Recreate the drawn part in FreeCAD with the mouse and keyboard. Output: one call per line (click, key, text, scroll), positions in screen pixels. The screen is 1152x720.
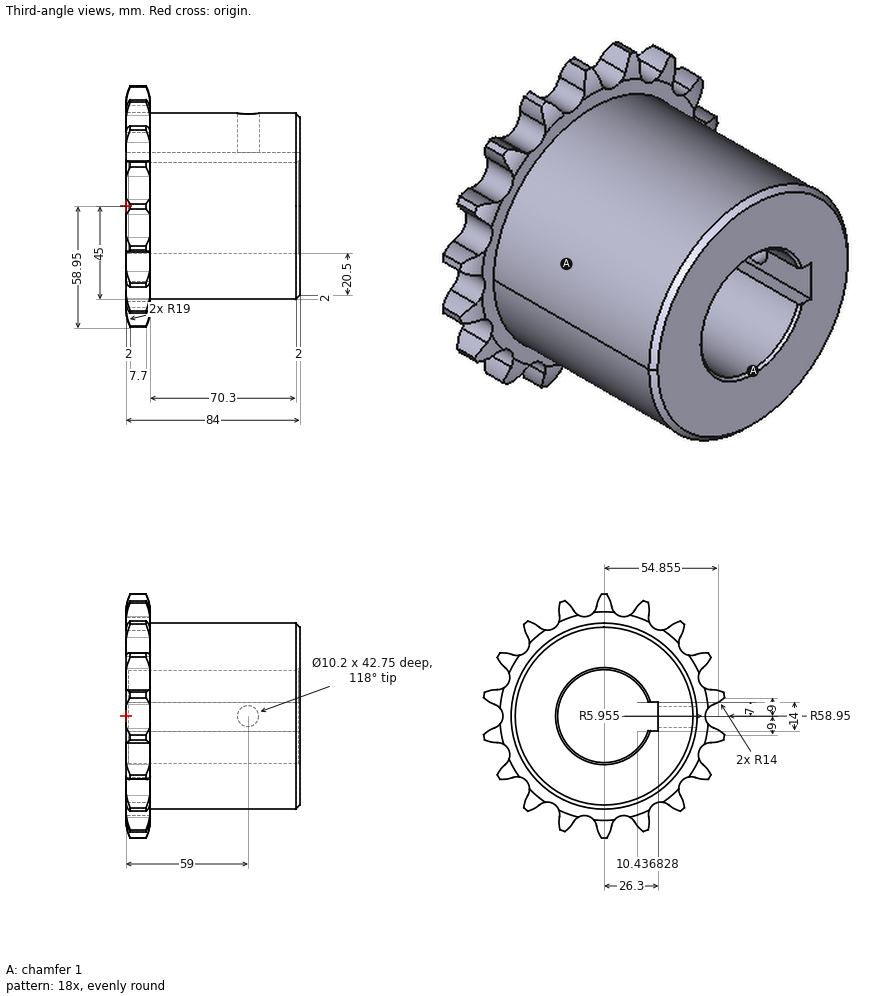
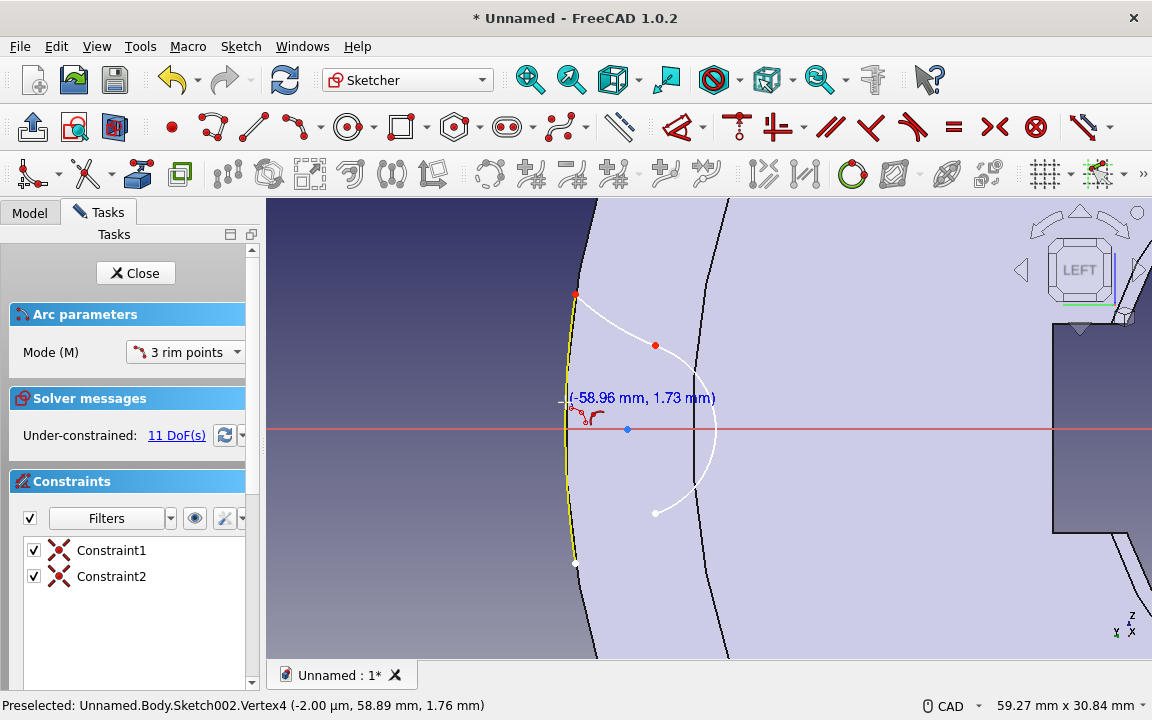
click(576, 564)
click(655, 514)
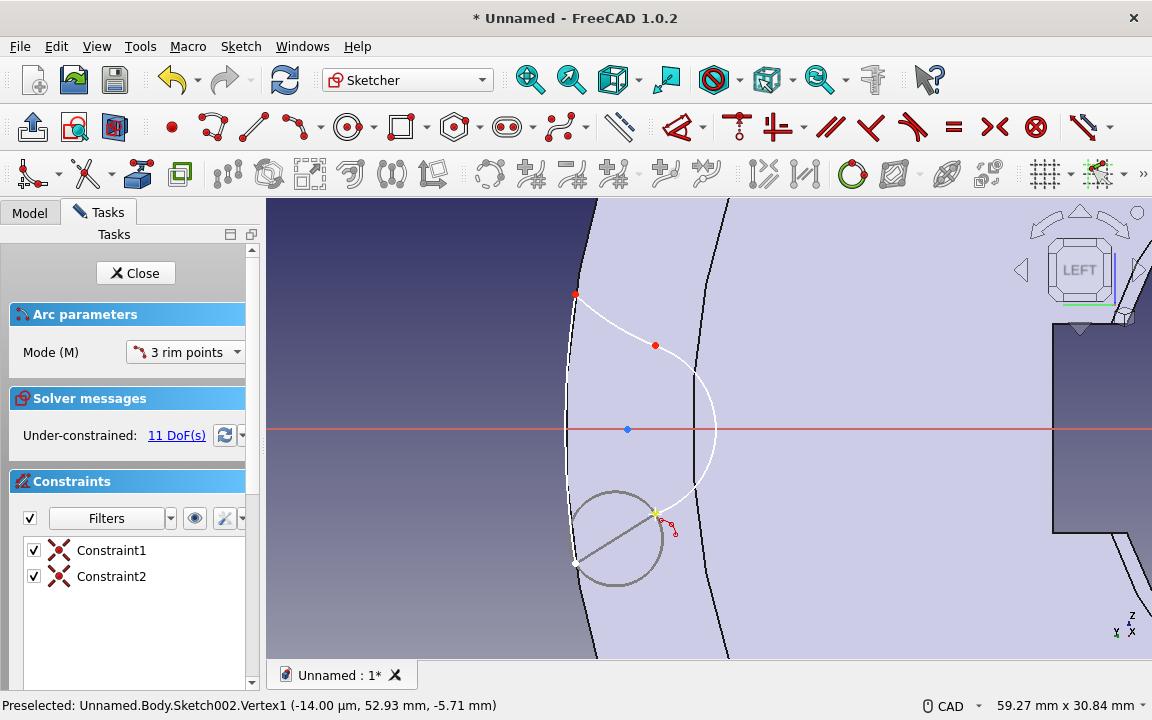
scroll(613, 533, up, 6)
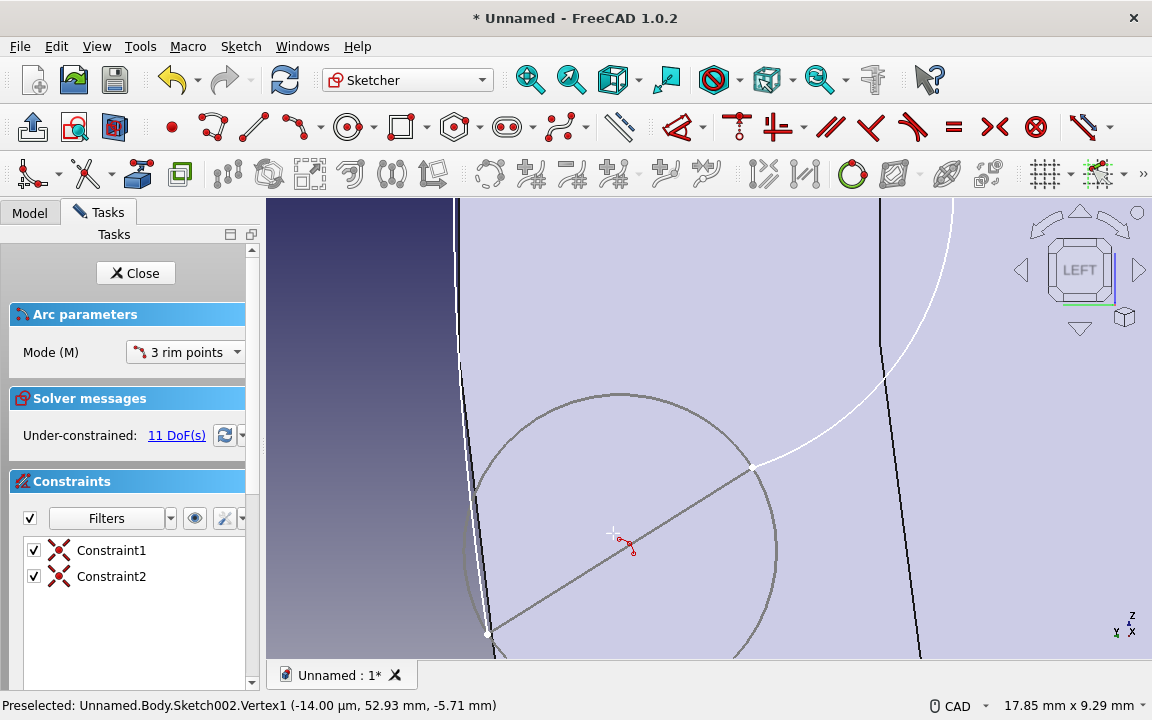
click(612, 532)
key(Escape)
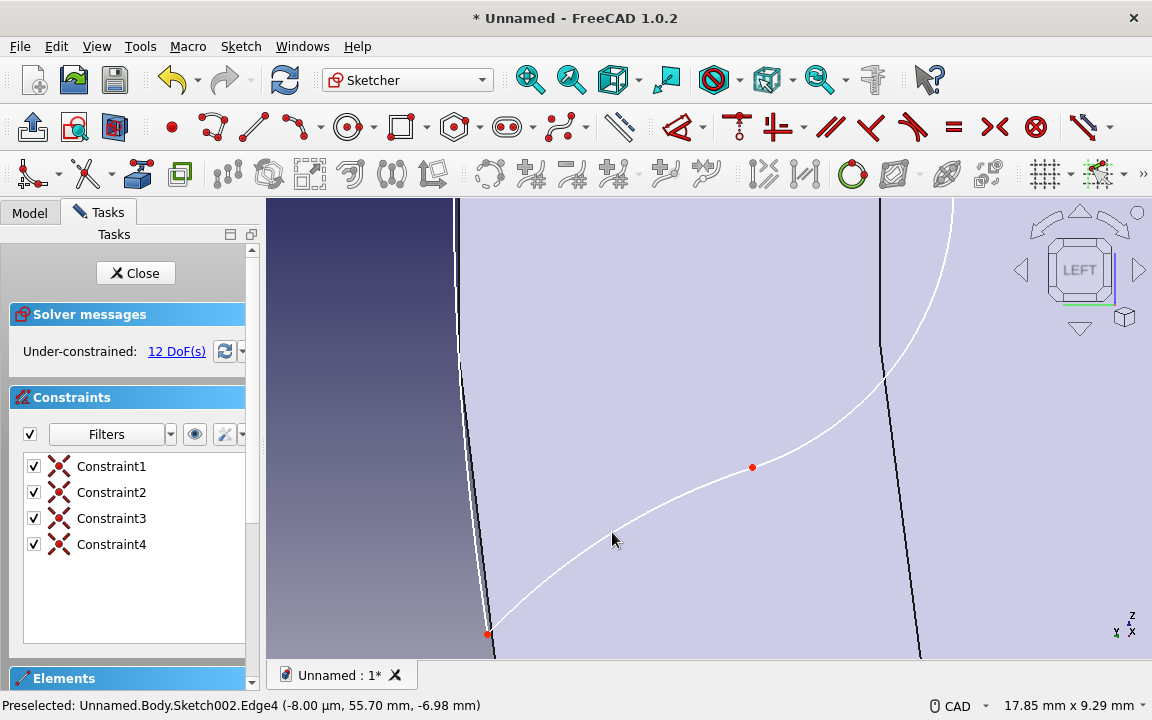
click(918, 330)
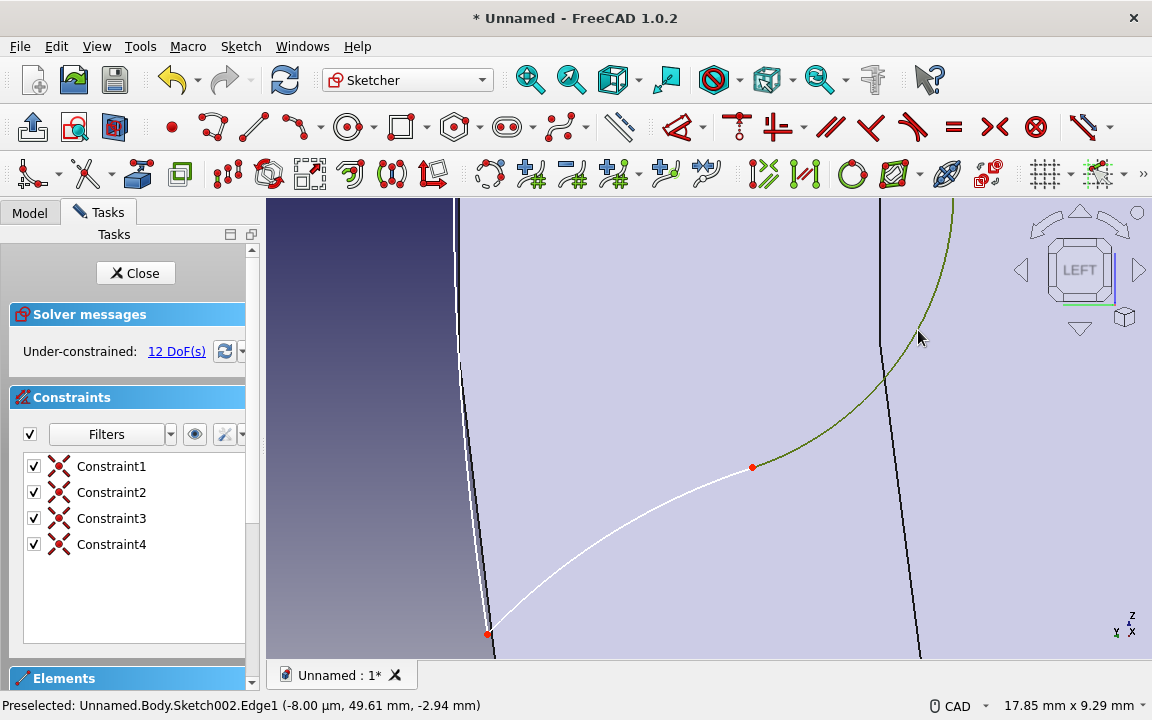
scroll(613, 534, down, 6)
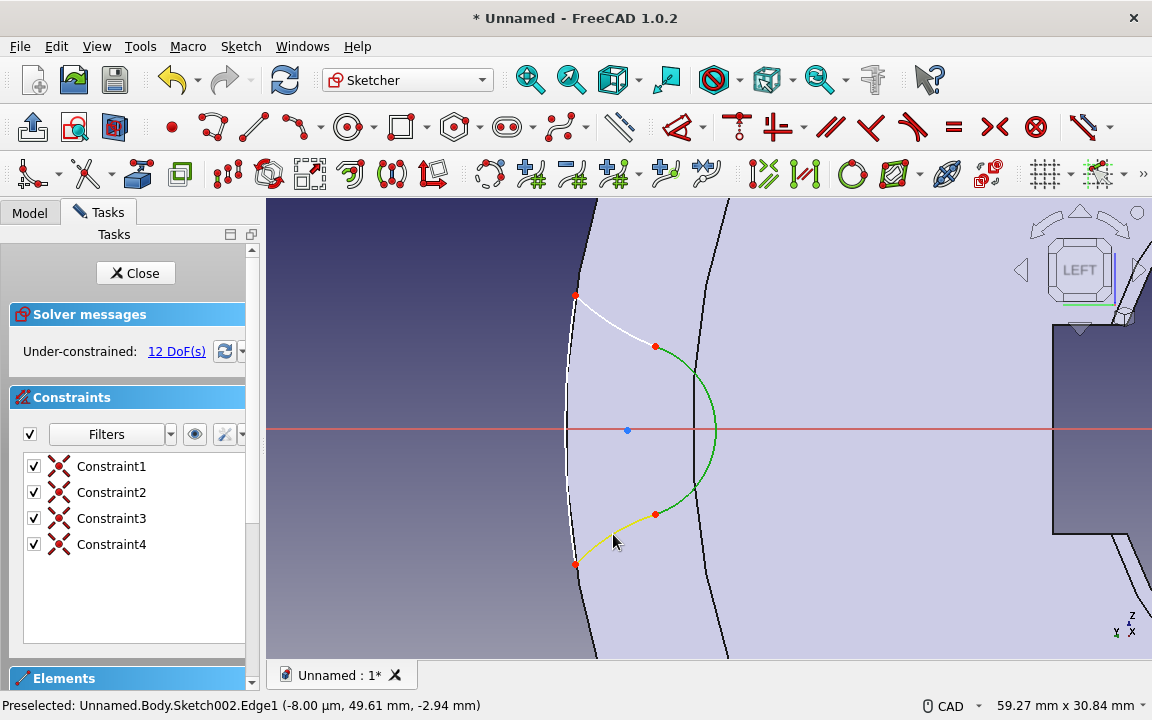
click(597, 314)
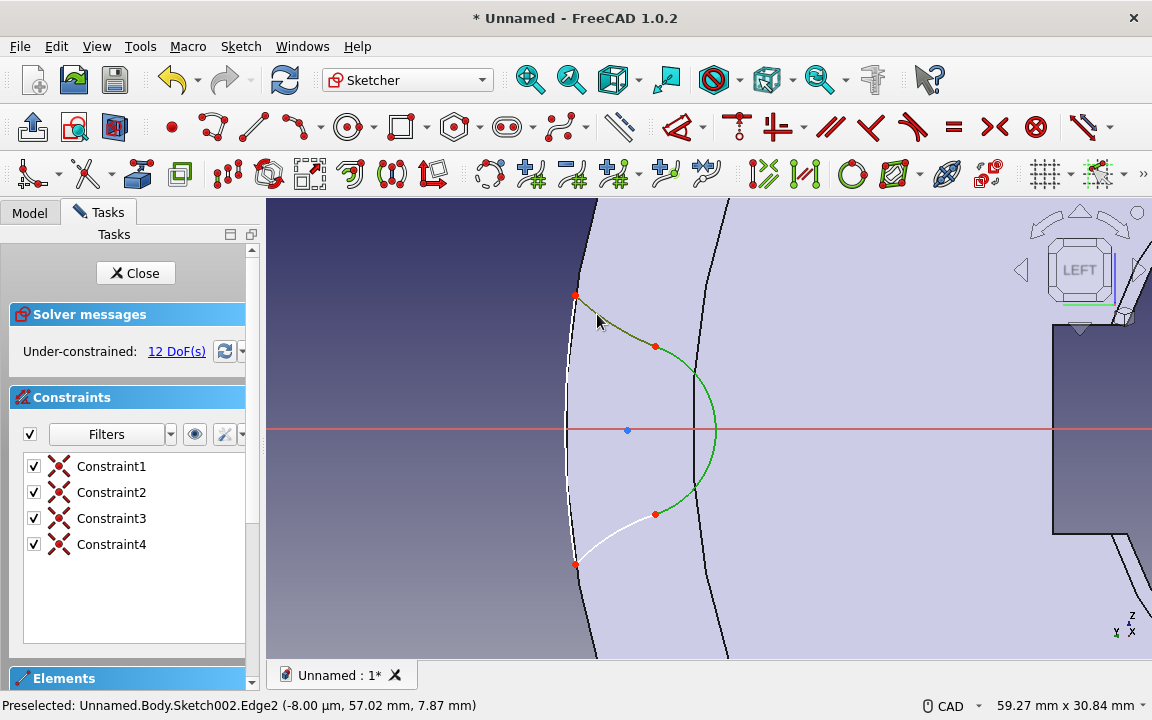
key(t)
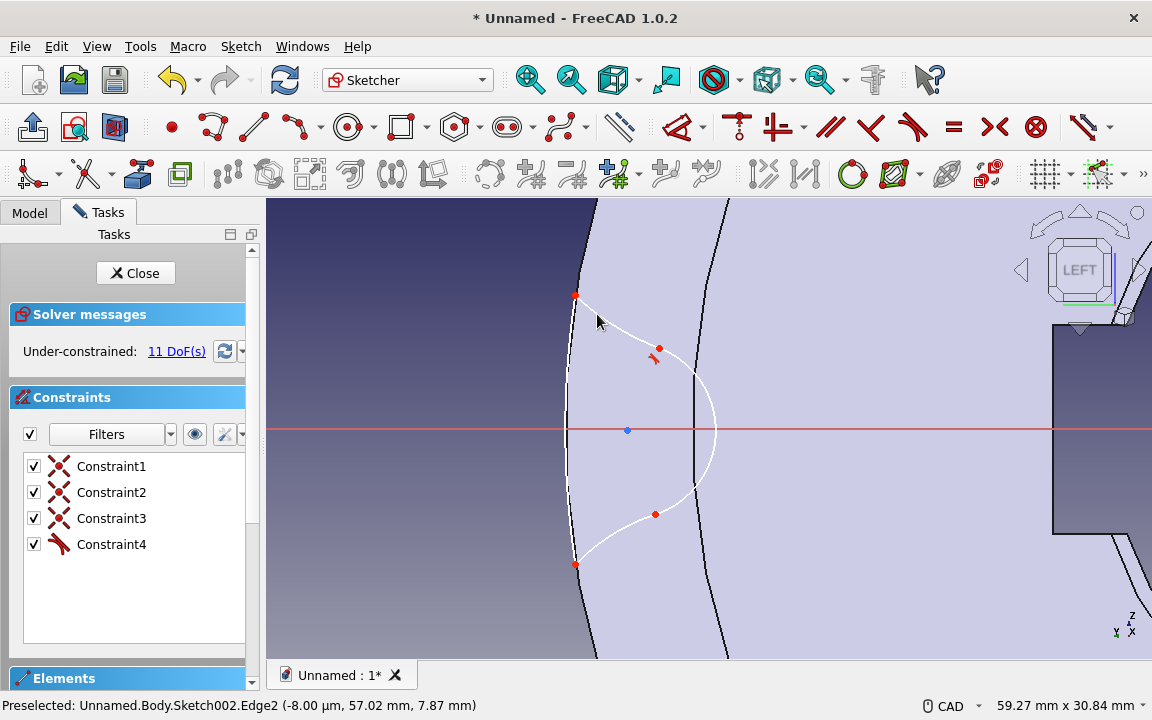
click(704, 474)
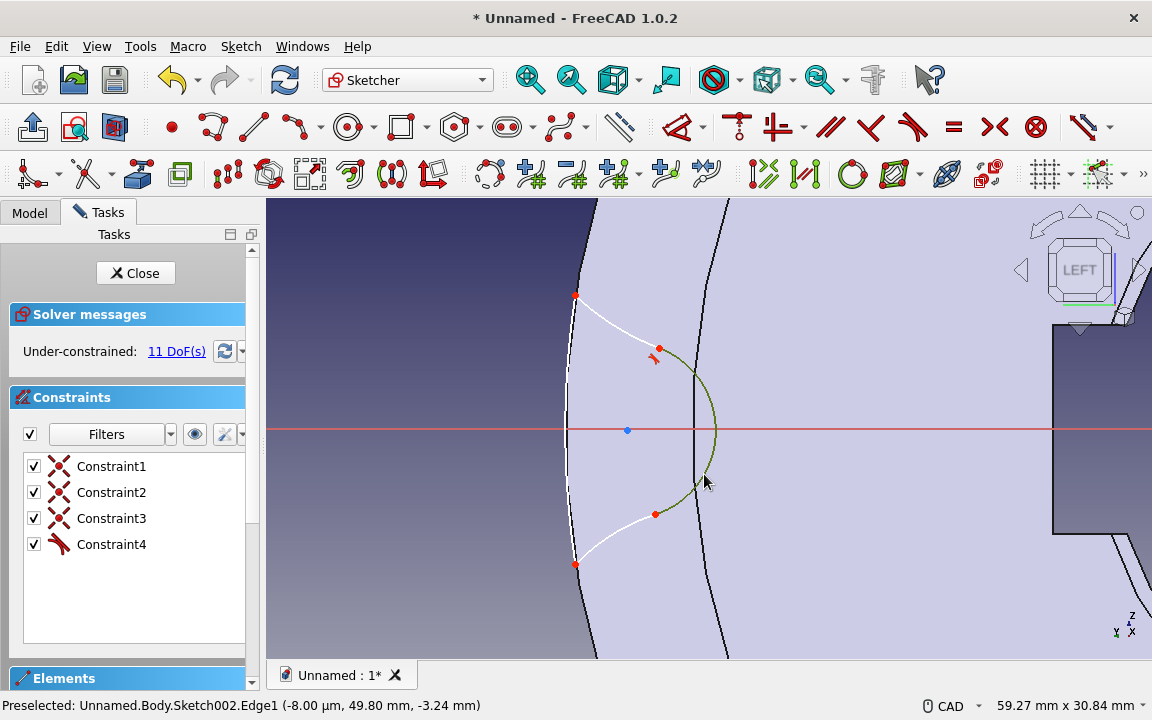
click(629, 525)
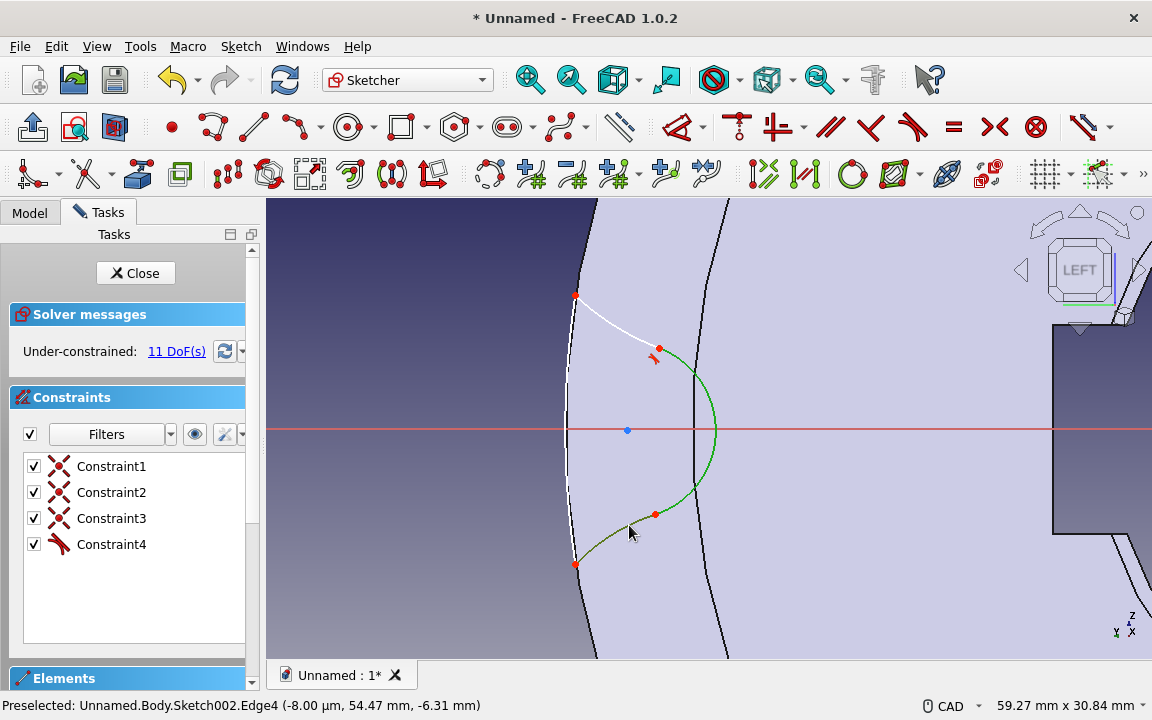
click(913, 128)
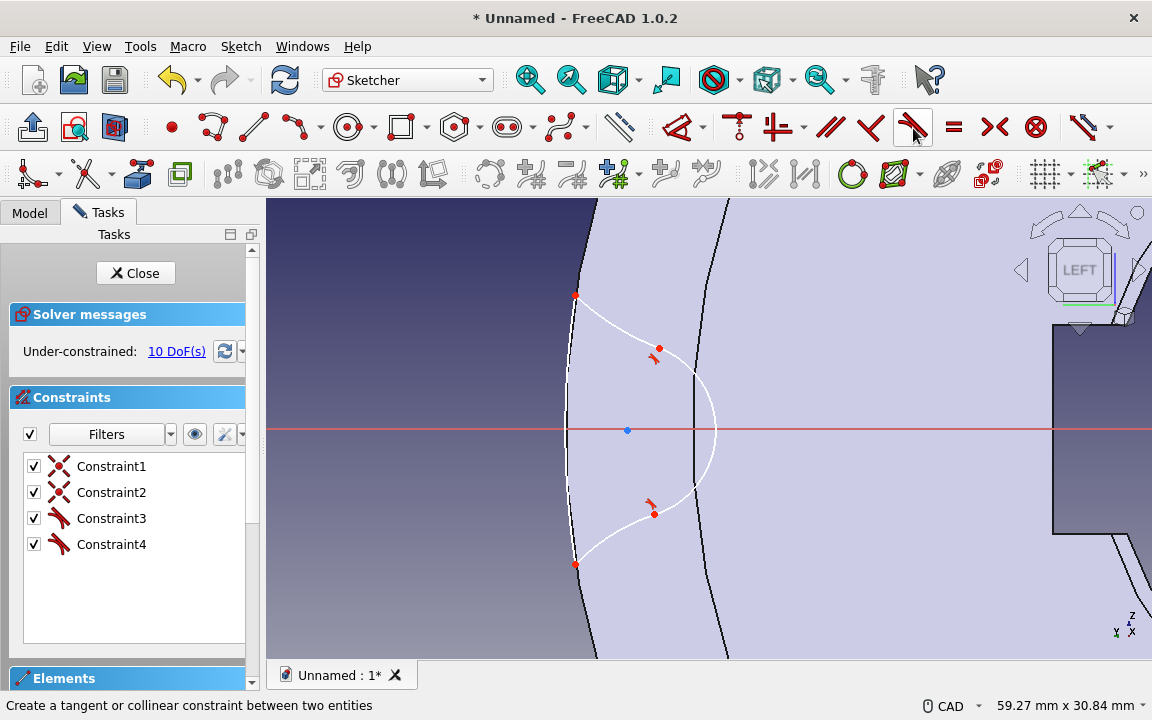
scroll(294, 428, down, 3)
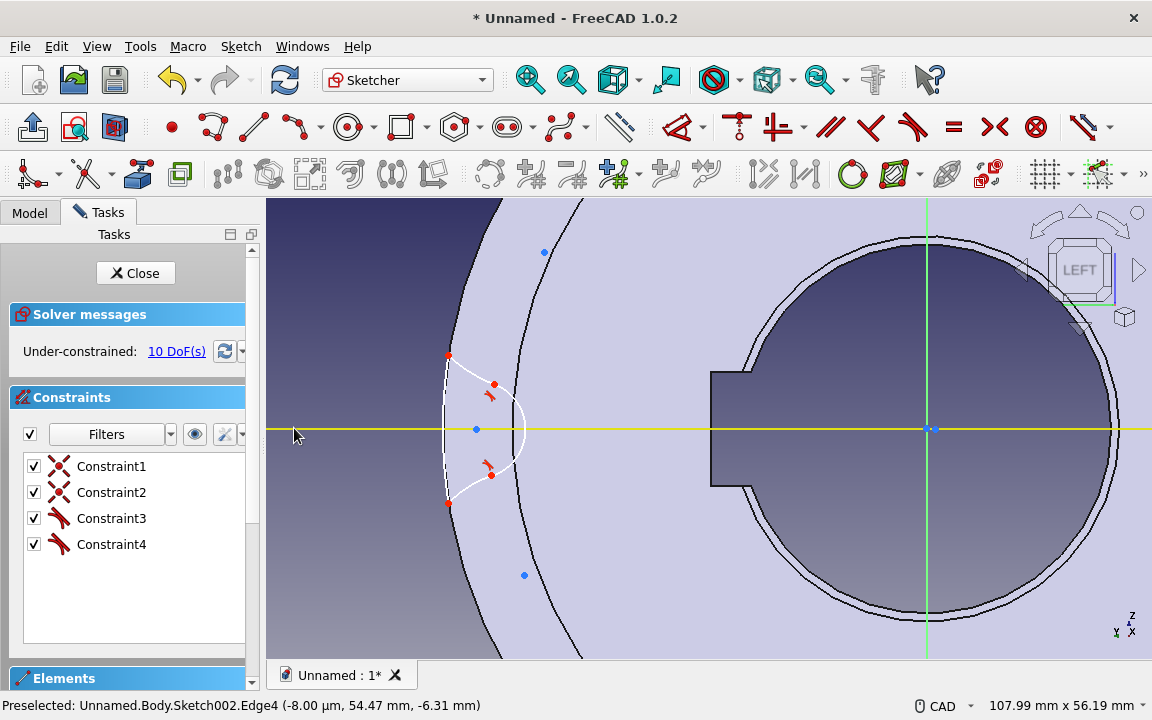
drag(917, 419, 946, 439)